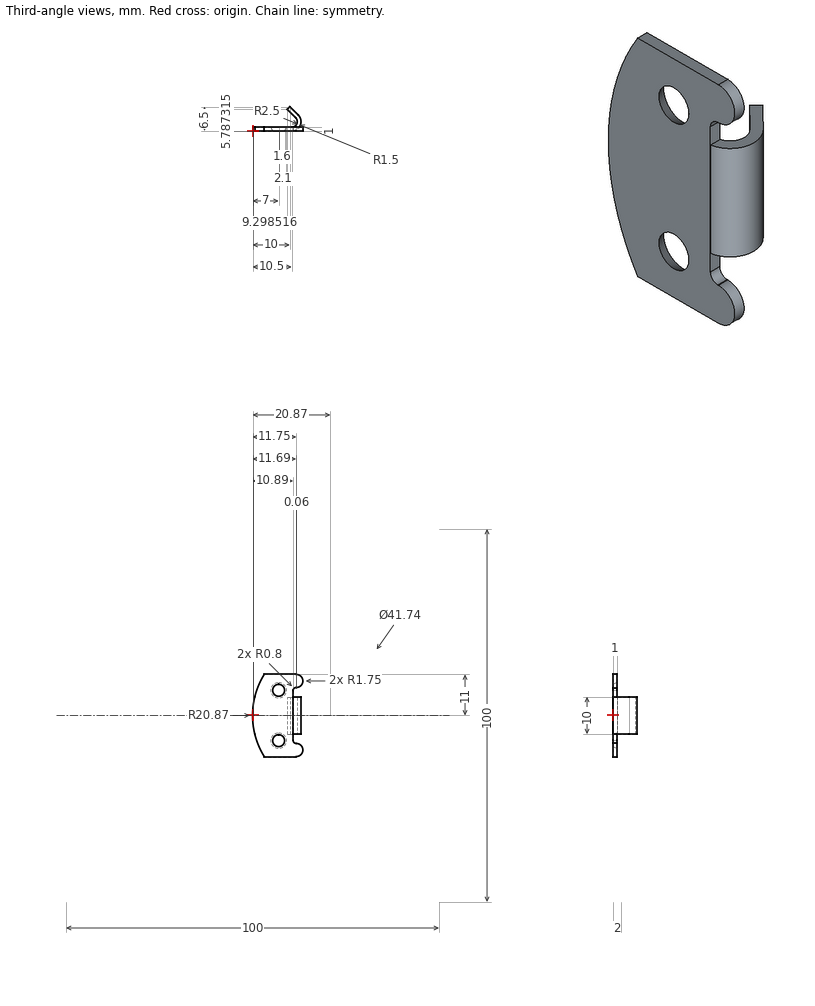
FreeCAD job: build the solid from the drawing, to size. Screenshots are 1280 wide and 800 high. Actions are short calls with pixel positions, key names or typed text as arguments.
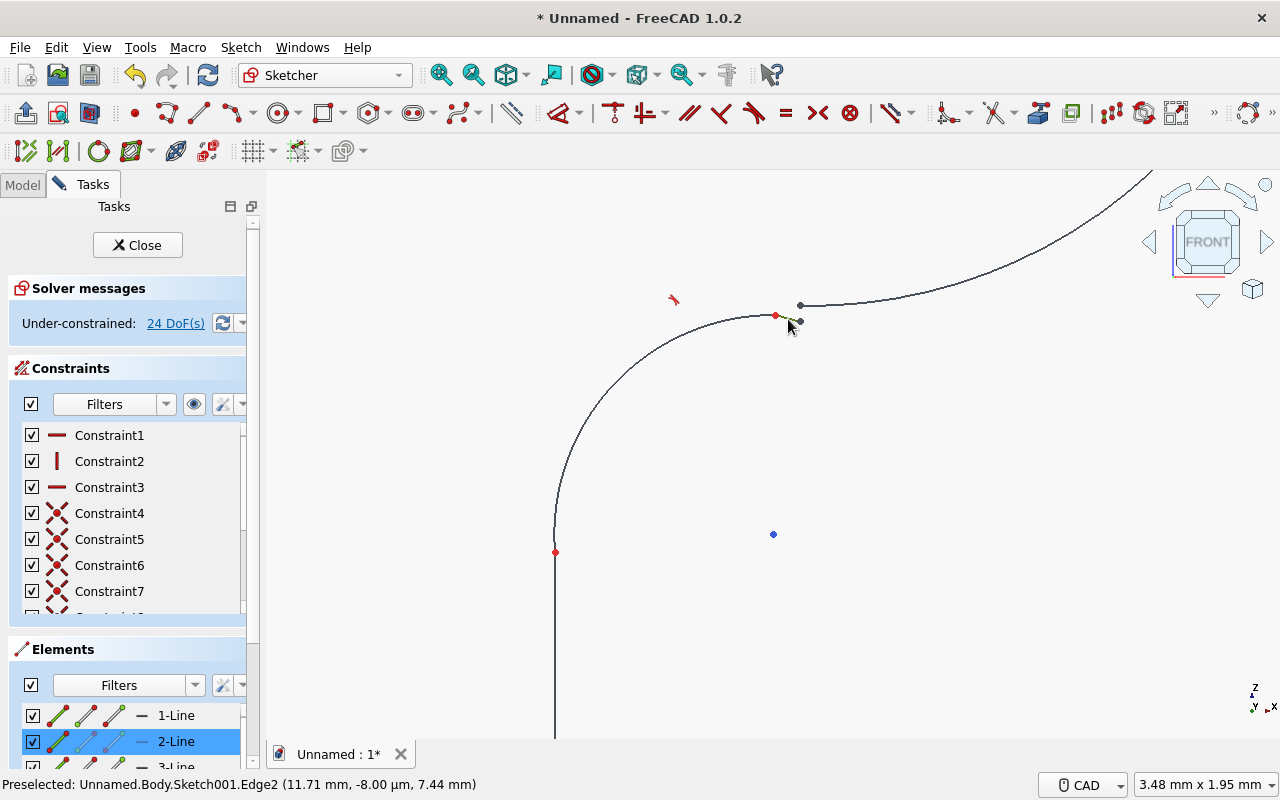
scroll(792, 323, down, 14)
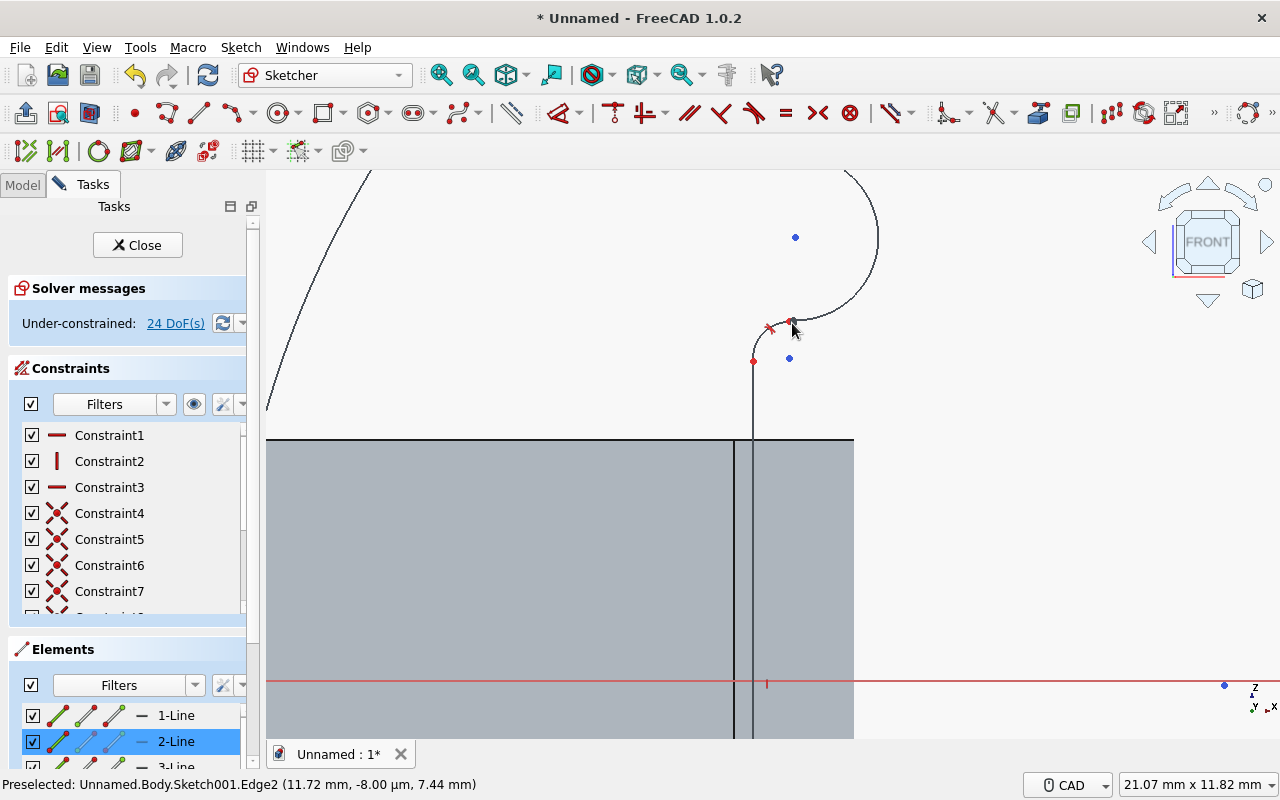
scroll(785, 324, up, 4)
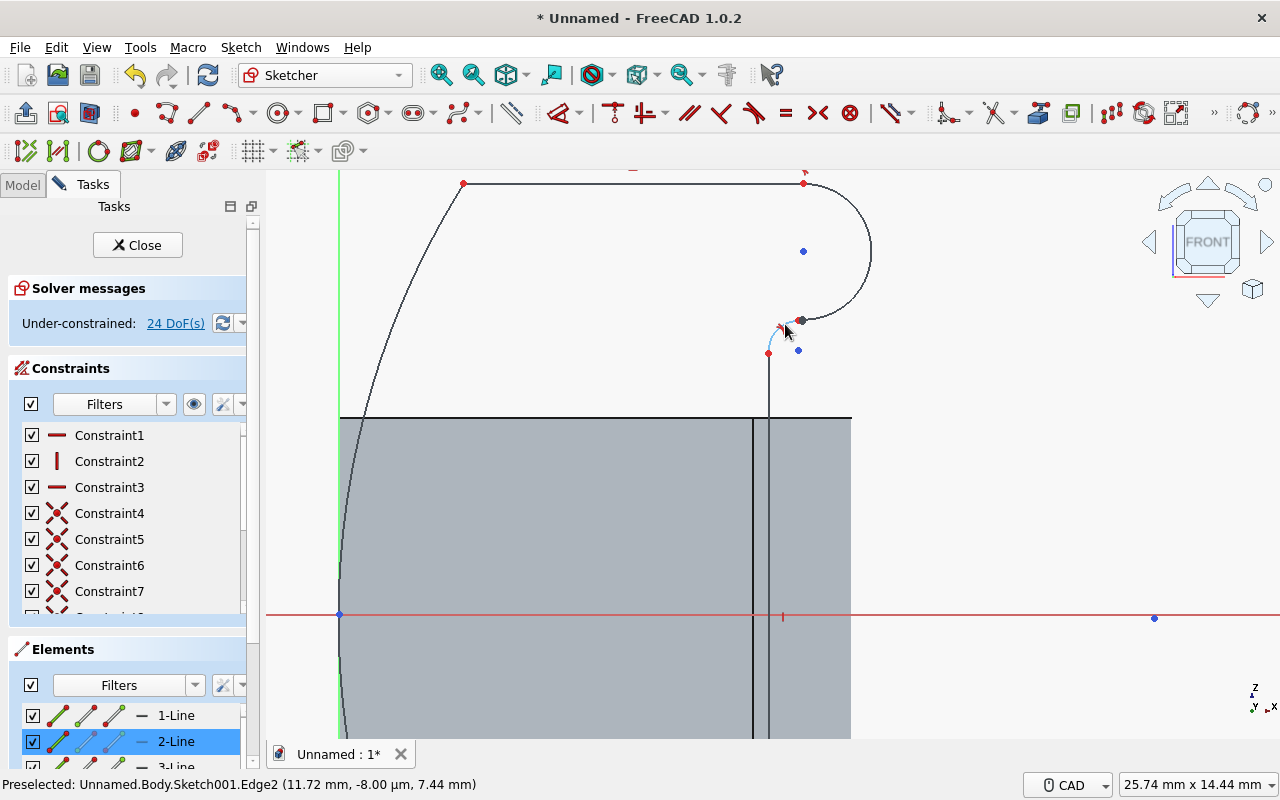
click(771, 339)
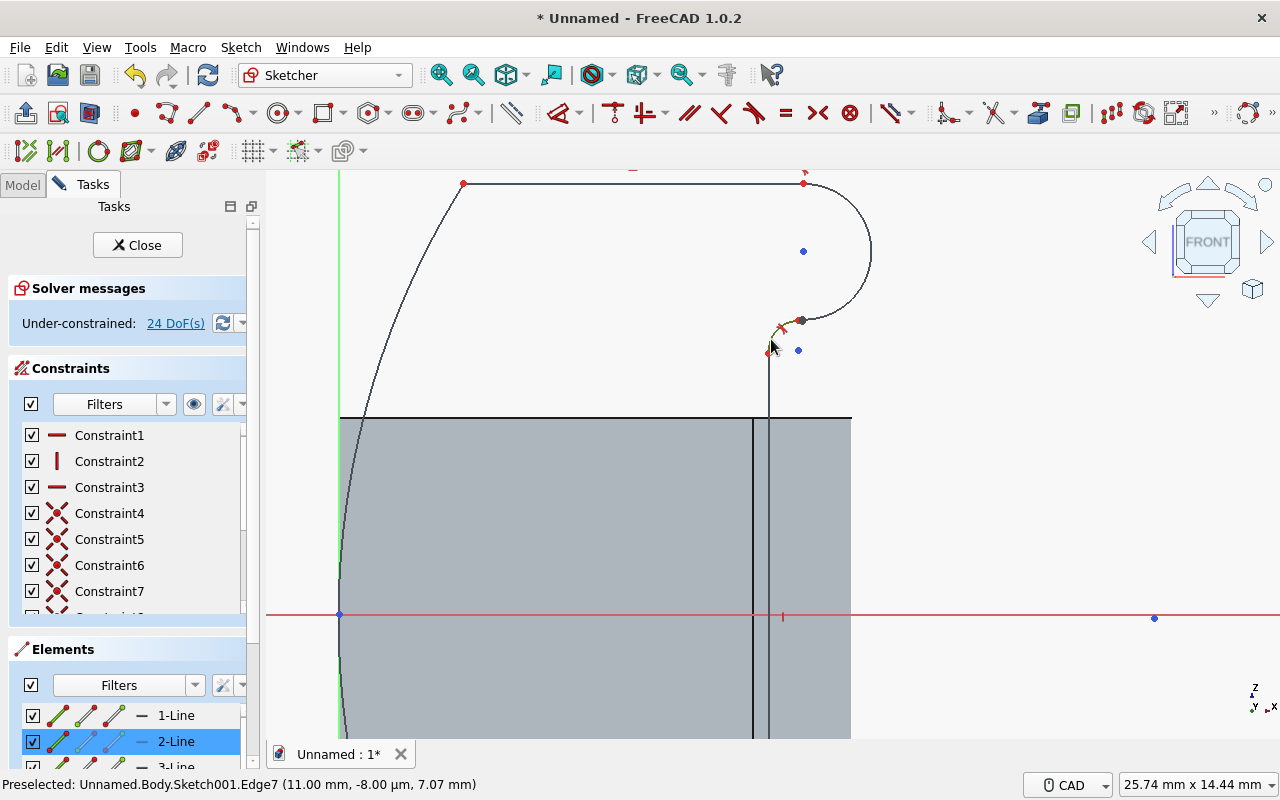
click(754, 114)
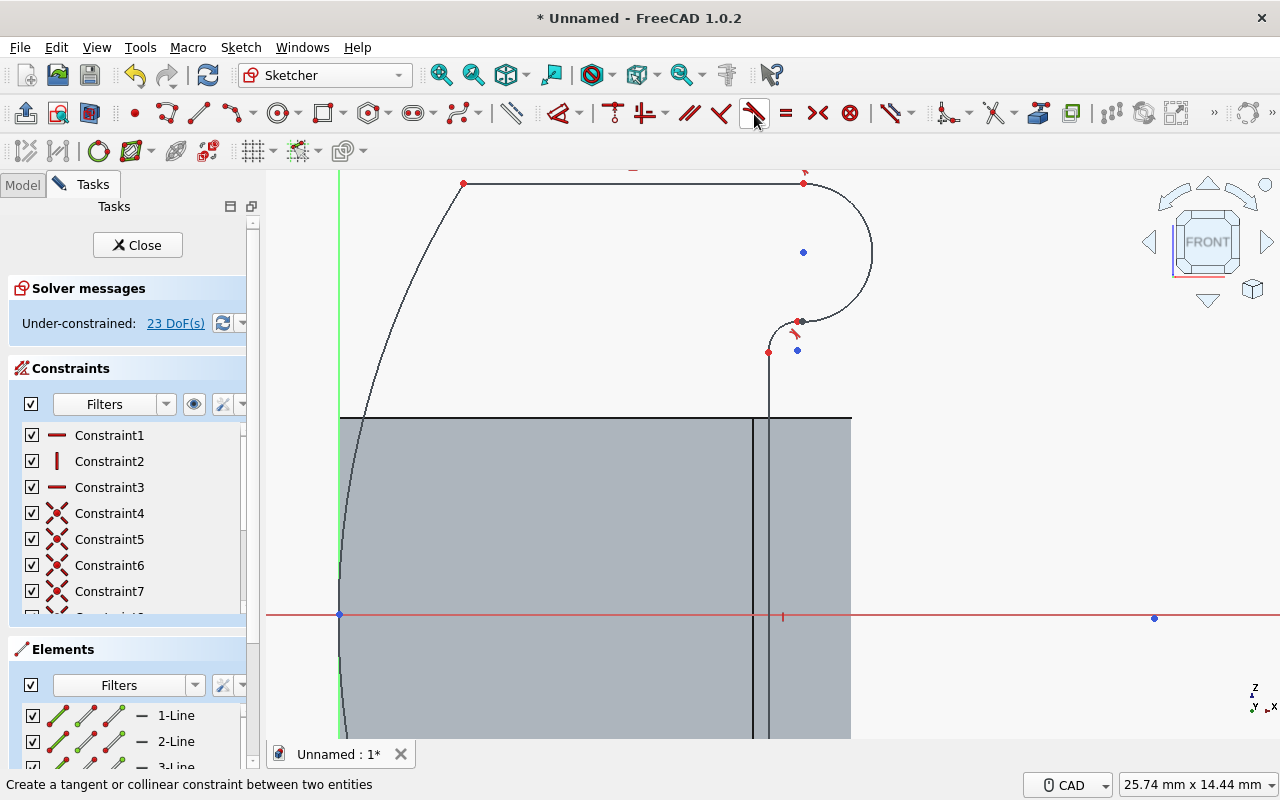
click(769, 511)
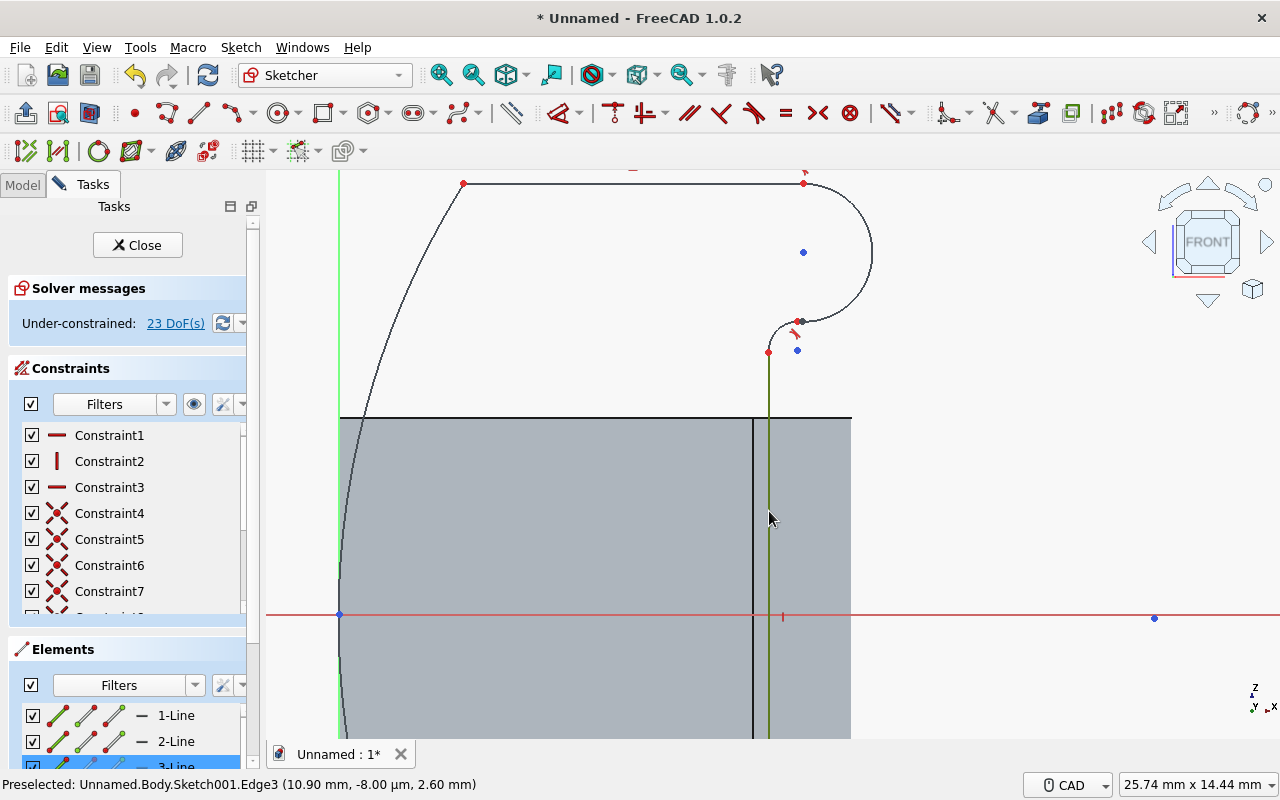
click(784, 325)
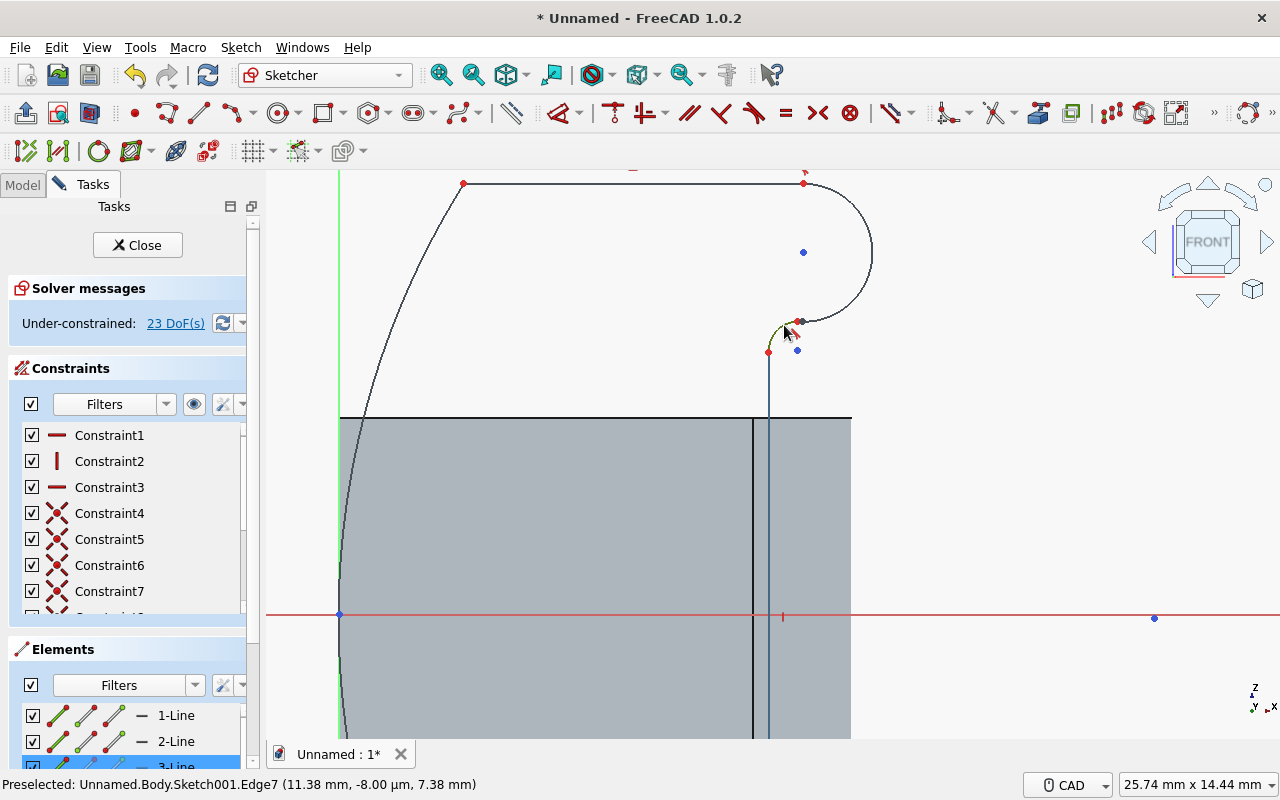
key(t)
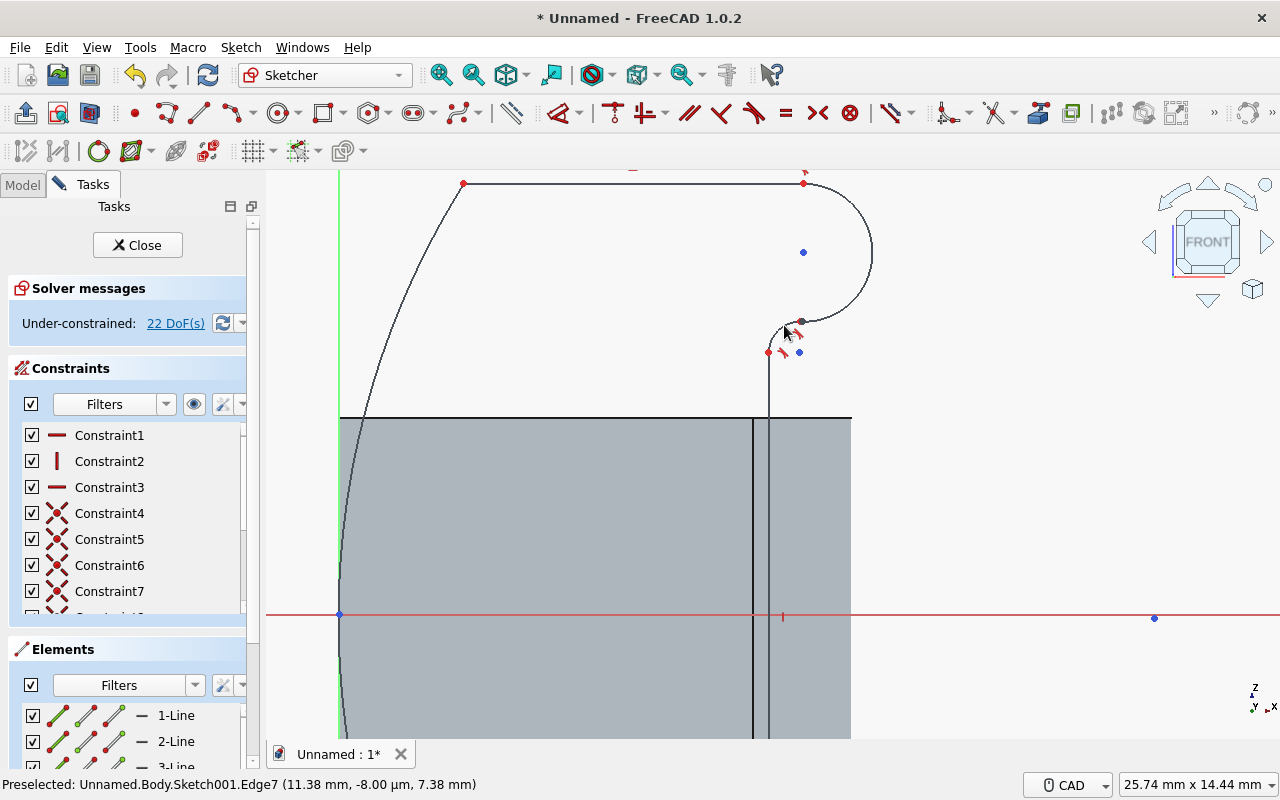
click(769, 511)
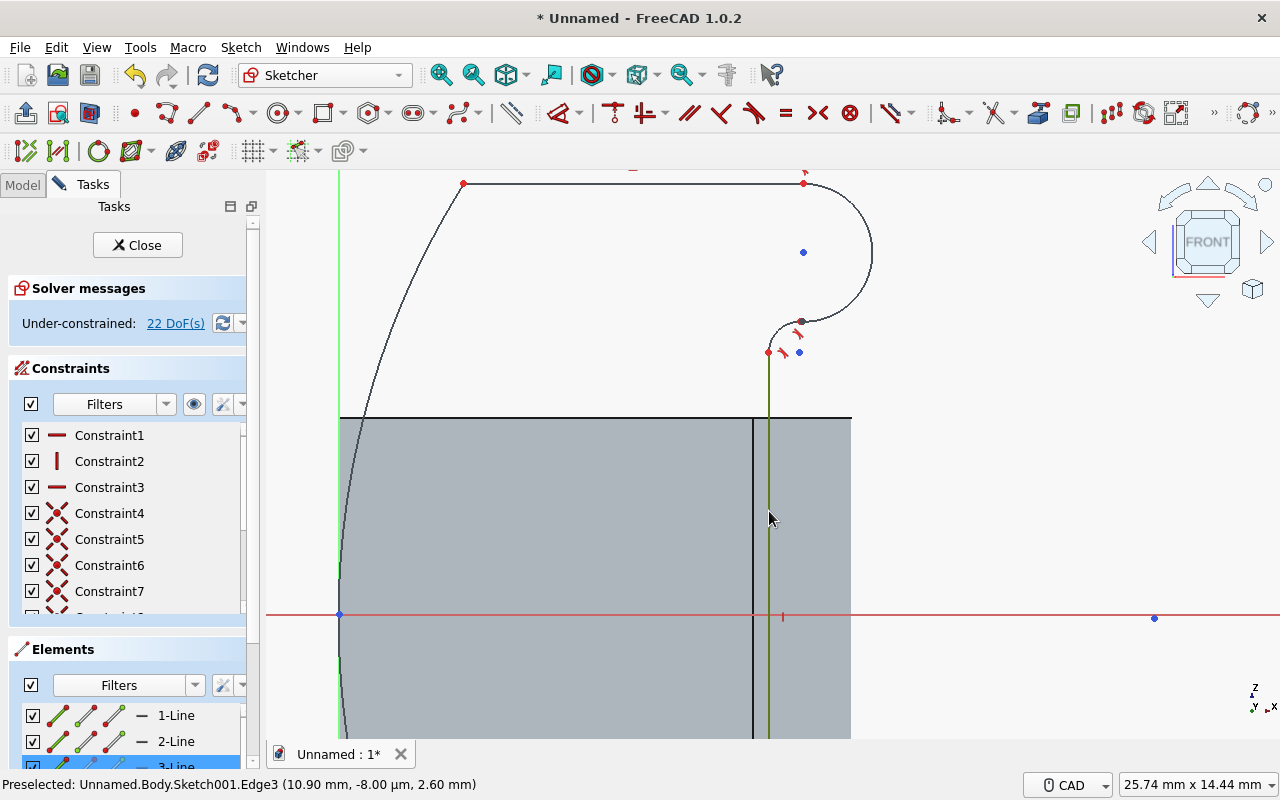
scroll(785, 324, down, 4)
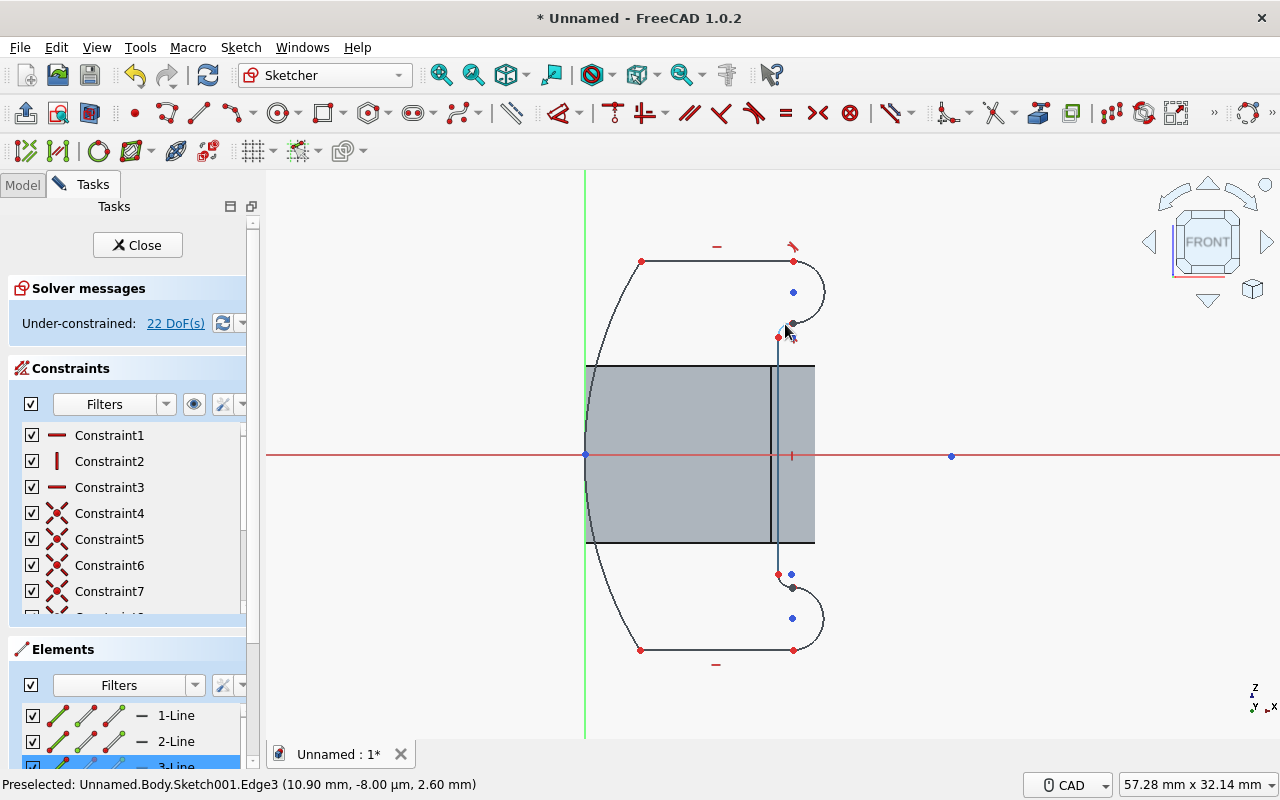
scroll(780, 580, up, 4)